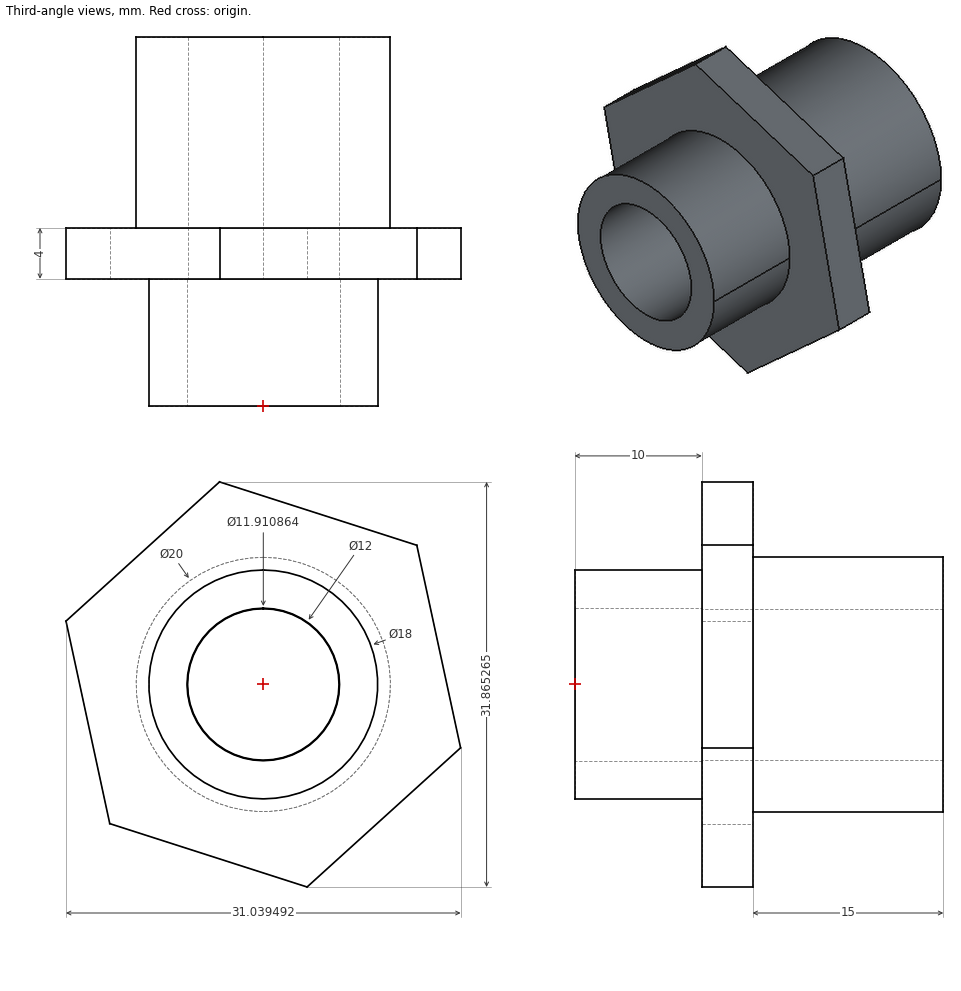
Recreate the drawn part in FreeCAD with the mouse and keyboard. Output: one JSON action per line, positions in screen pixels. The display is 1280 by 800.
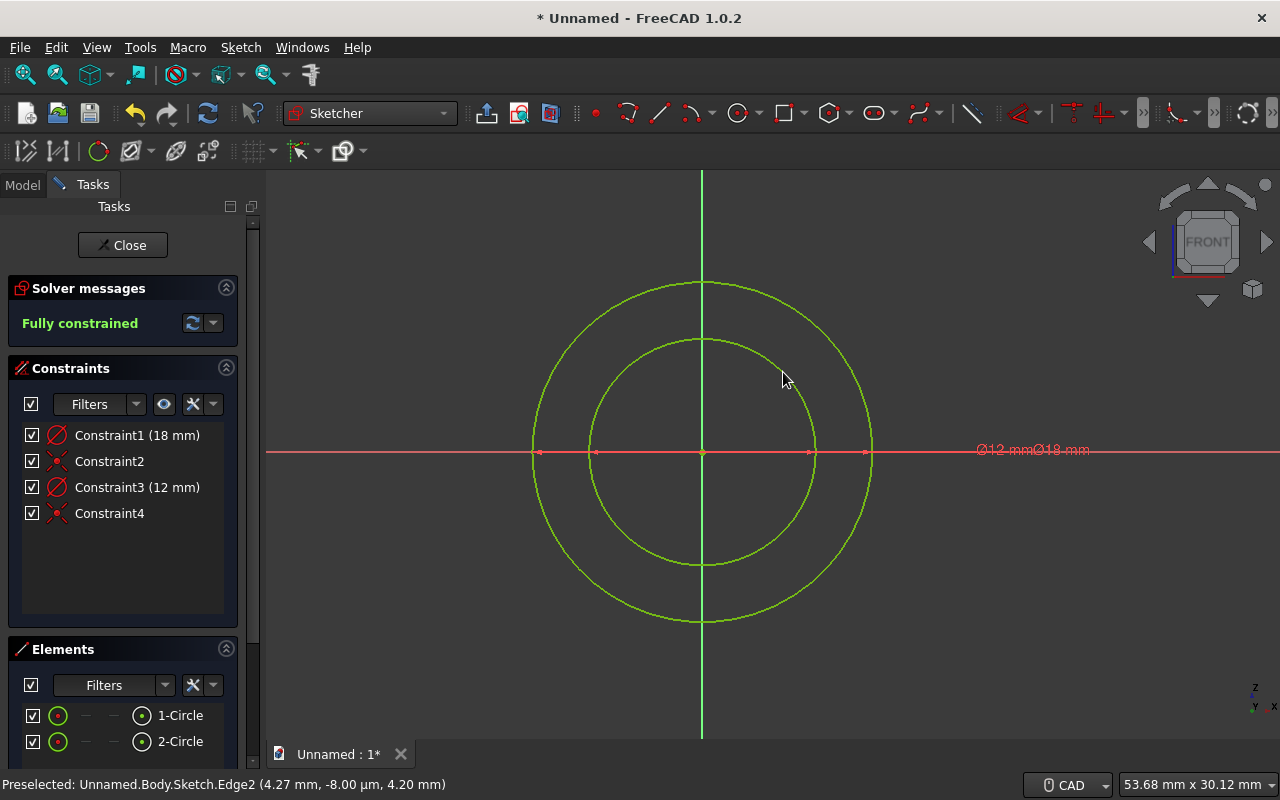
{"action": "left_click", "coordinate": [123, 245]}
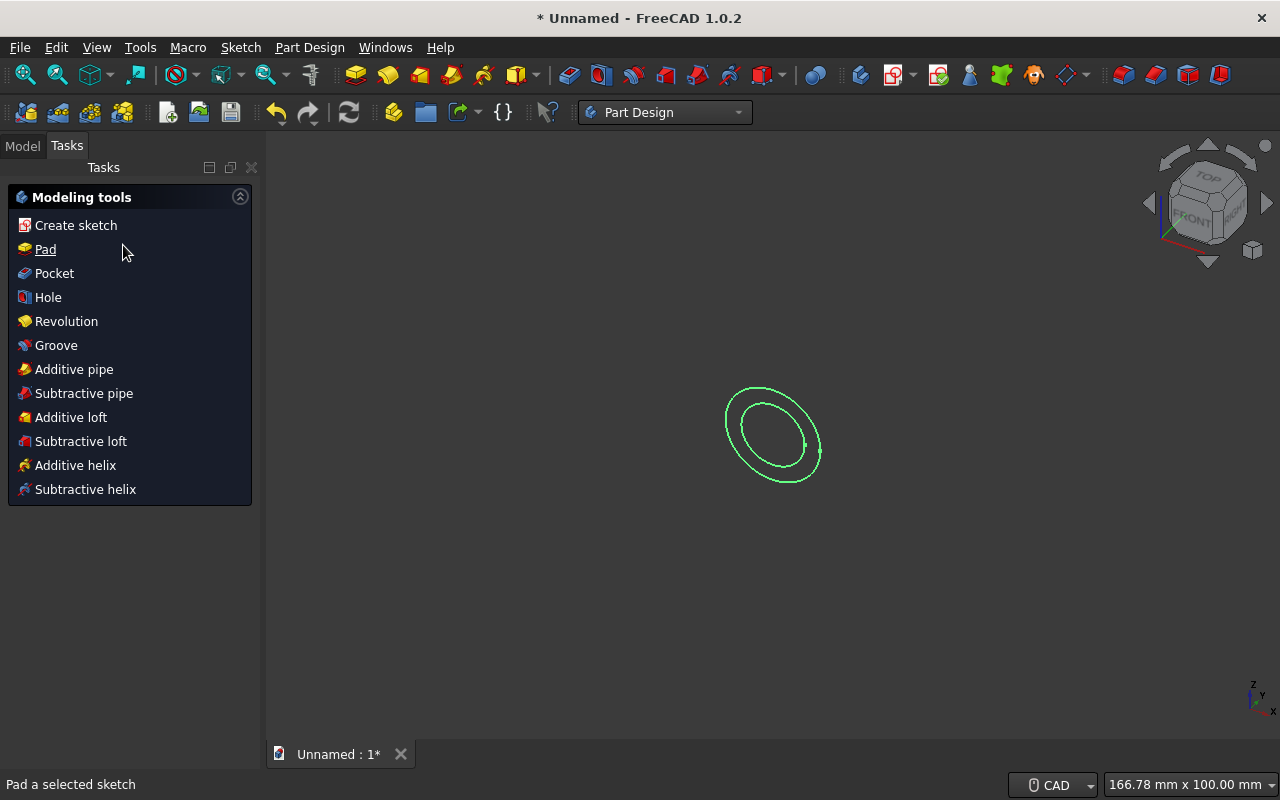
{"action": "left_click", "coordinate": [356, 76]}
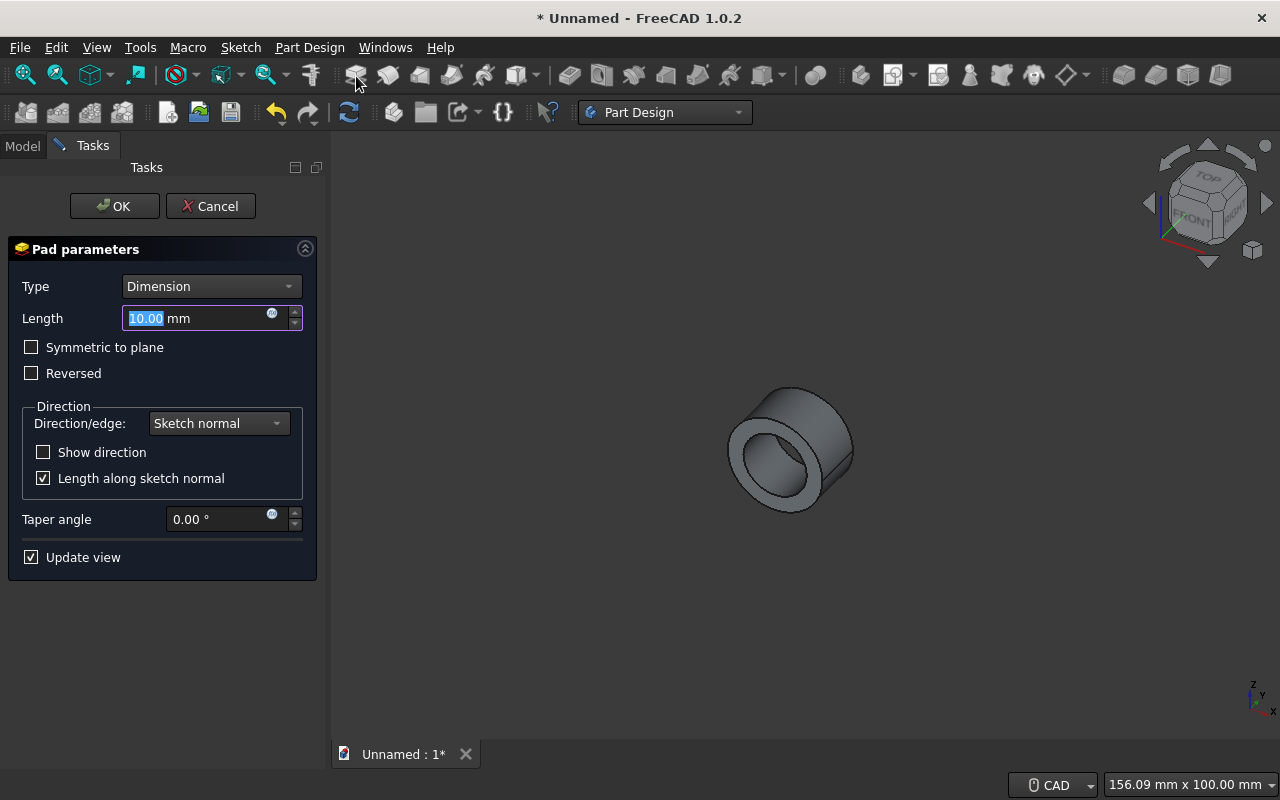
{"action": "type", "text": "10"}
{"action": "key", "text": "Tab"}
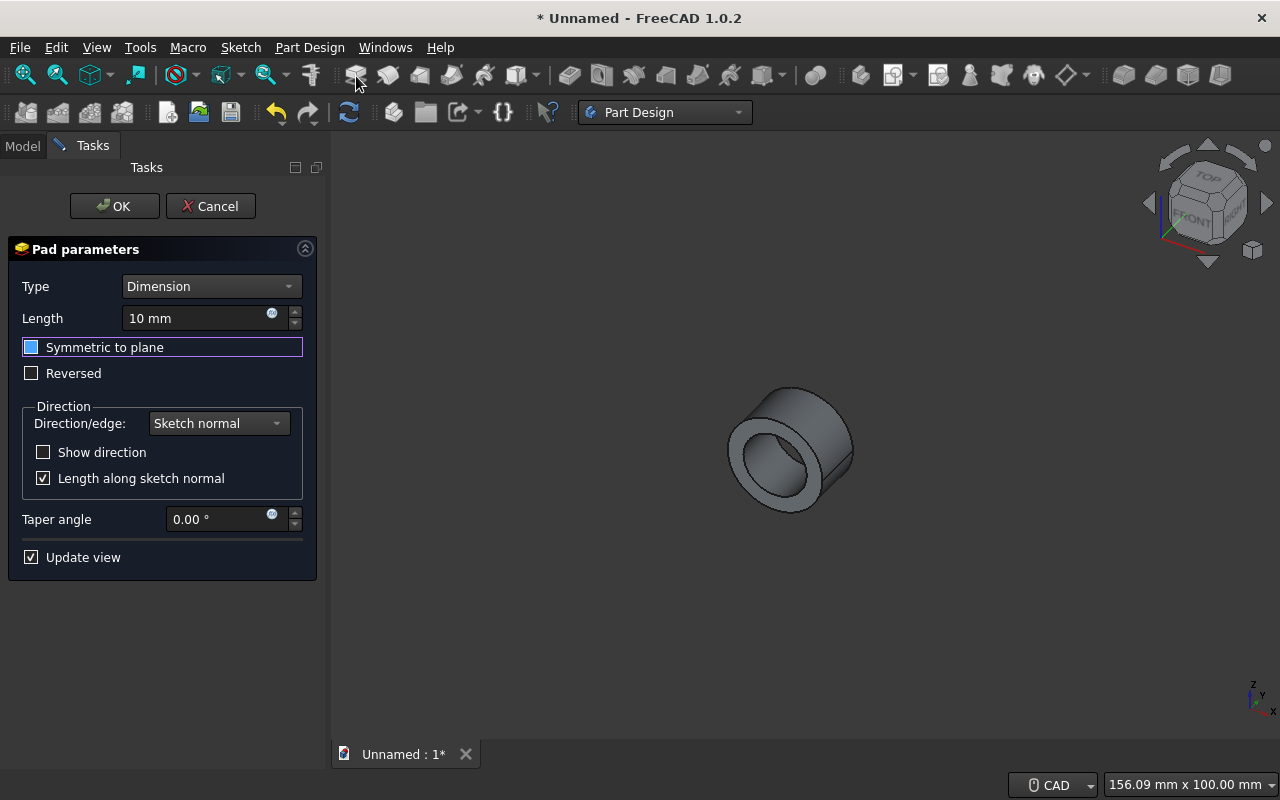
{"action": "left_click", "coordinate": [30, 373]}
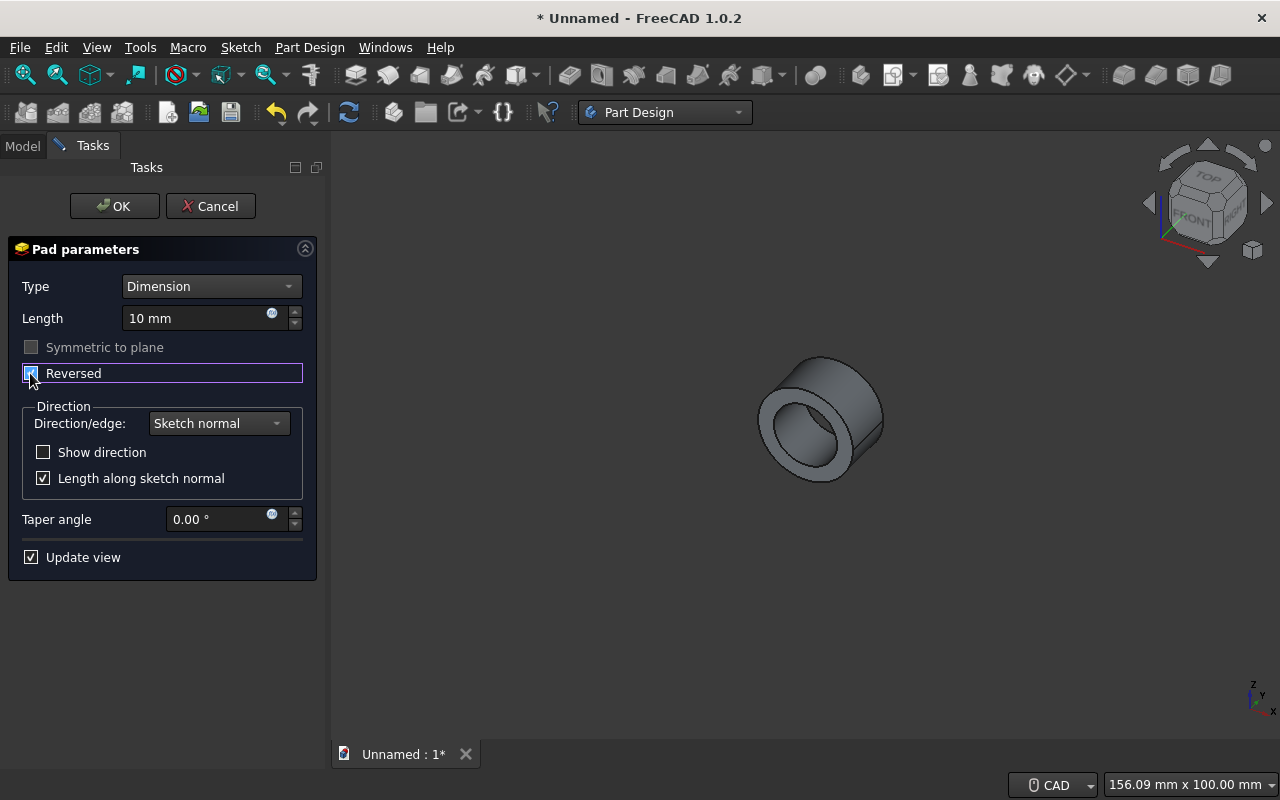
{"action": "left_click", "coordinate": [115, 206]}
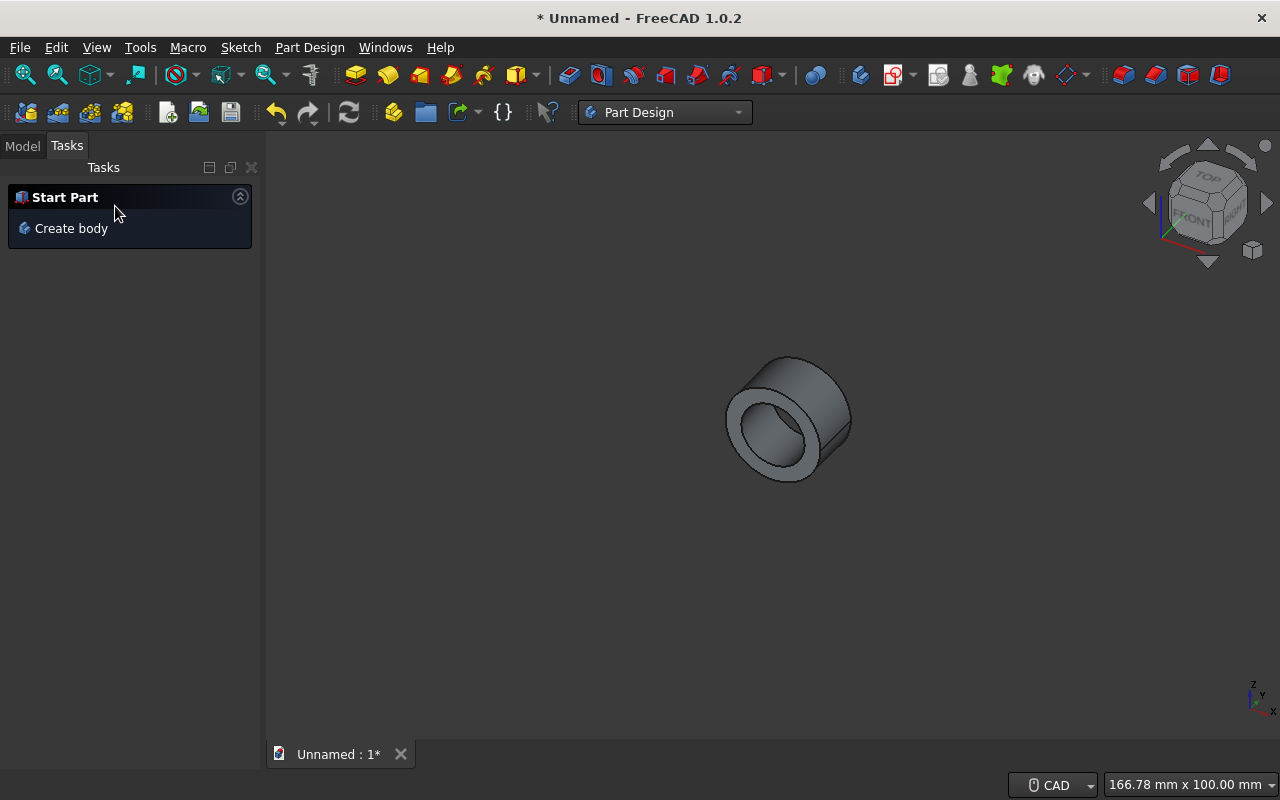
{"action": "left_click", "coordinate": [26, 76]}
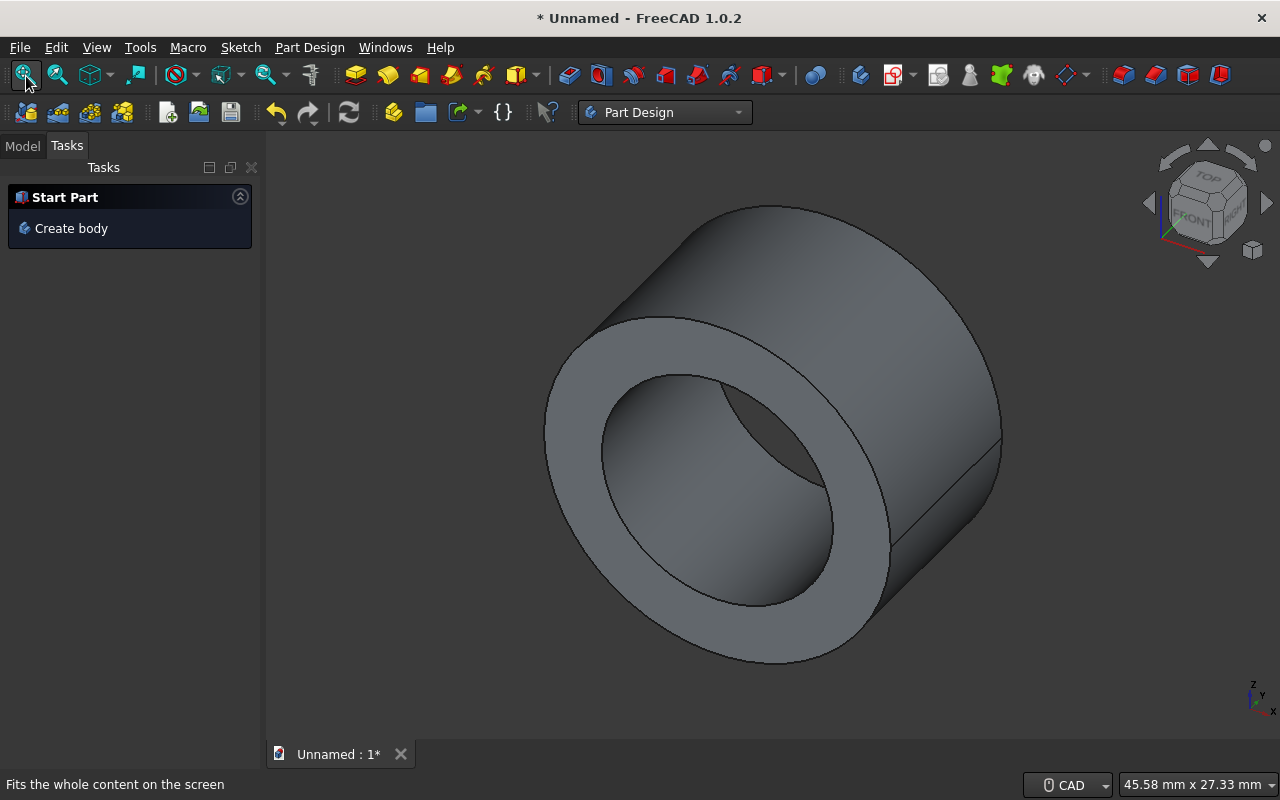
{"action": "left_click", "coordinate": [862, 76]}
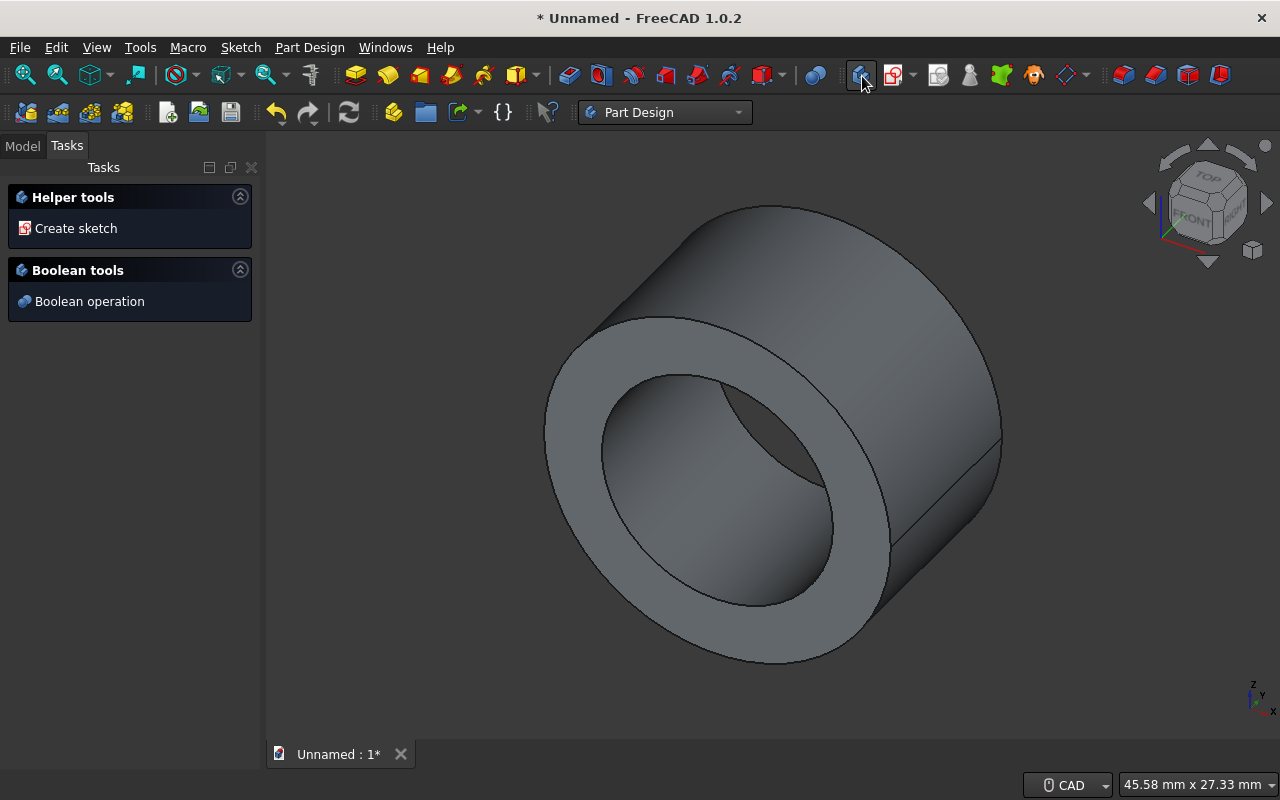
{"action": "left_click", "coordinate": [23, 145]}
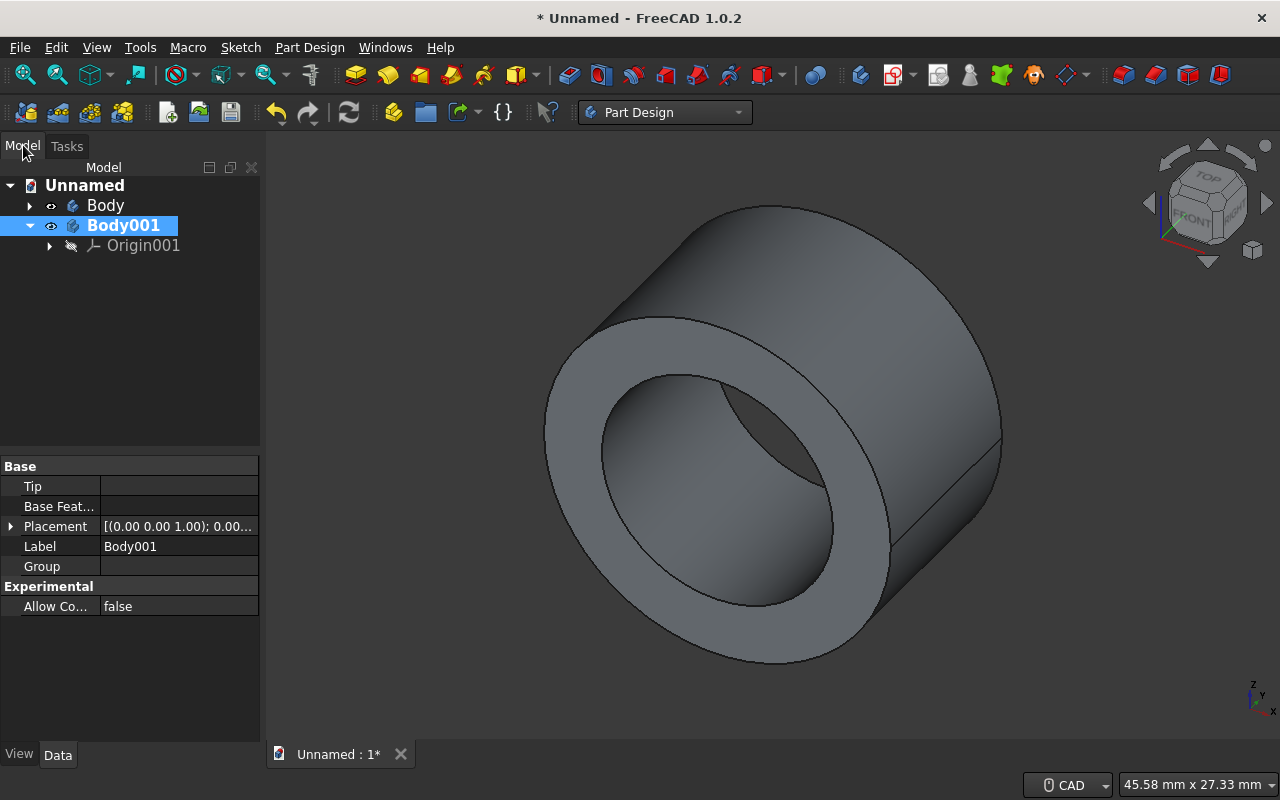
{"action": "left_click", "coordinate": [50, 246]}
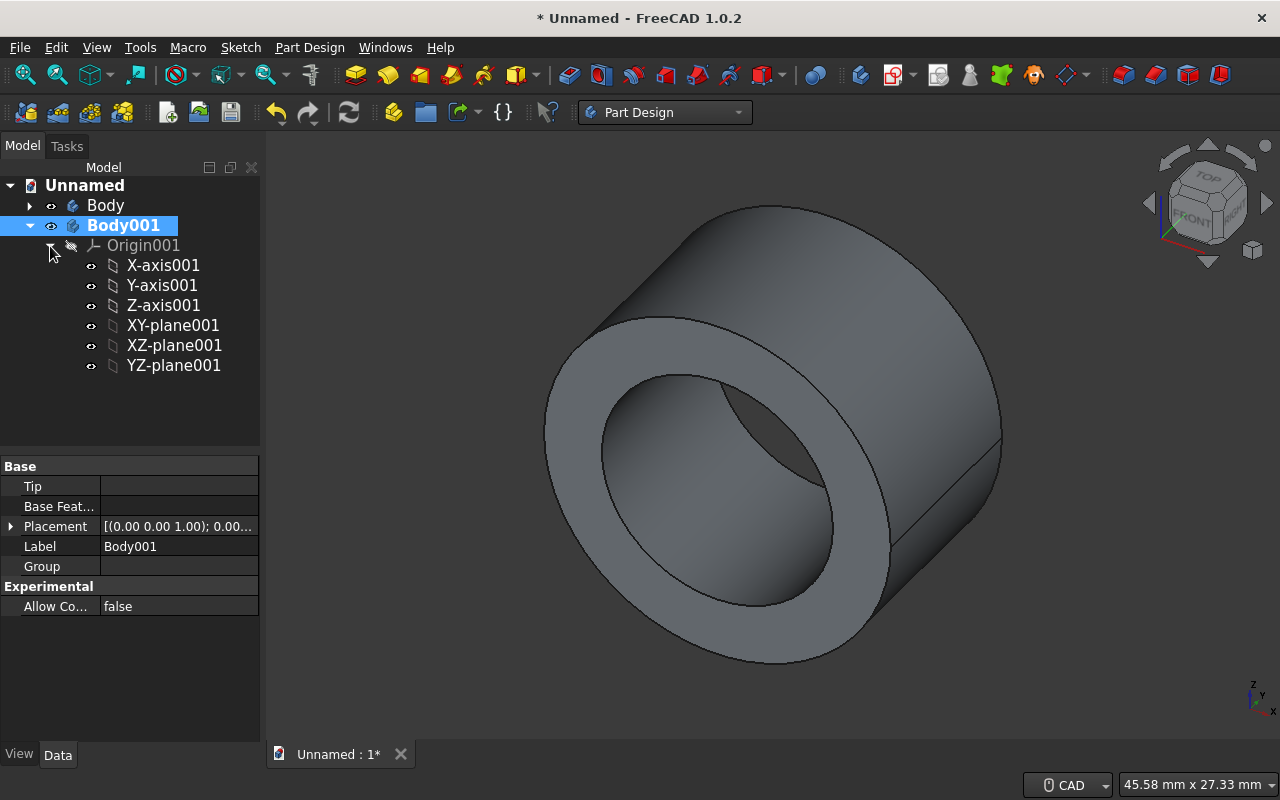
{"action": "left_click", "coordinate": [136, 346]}